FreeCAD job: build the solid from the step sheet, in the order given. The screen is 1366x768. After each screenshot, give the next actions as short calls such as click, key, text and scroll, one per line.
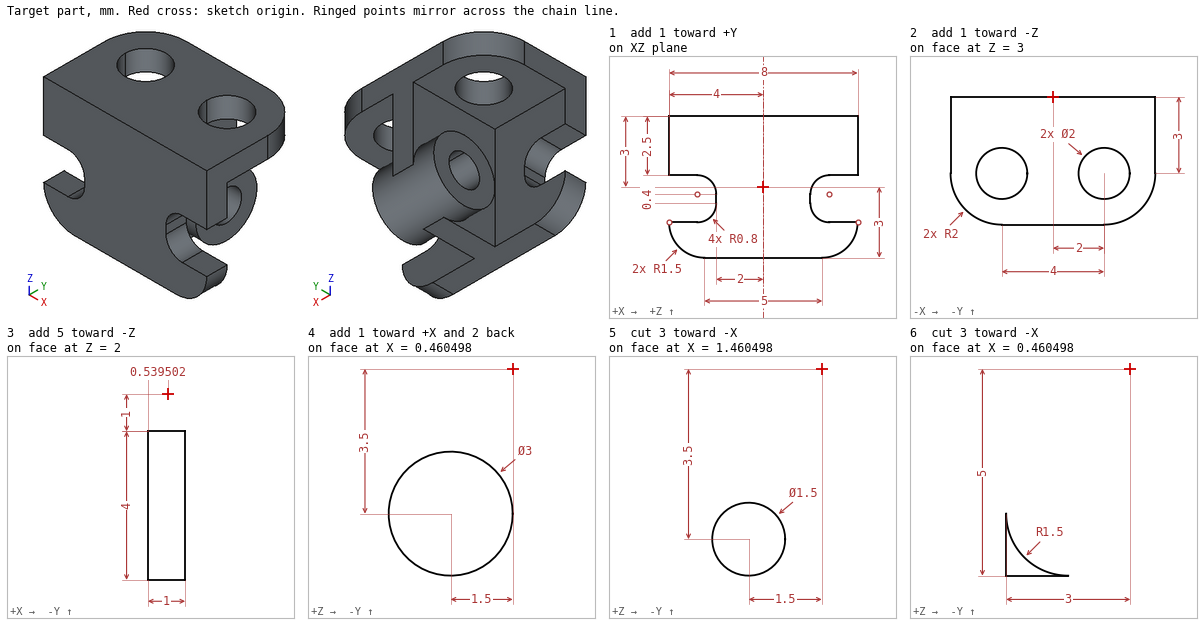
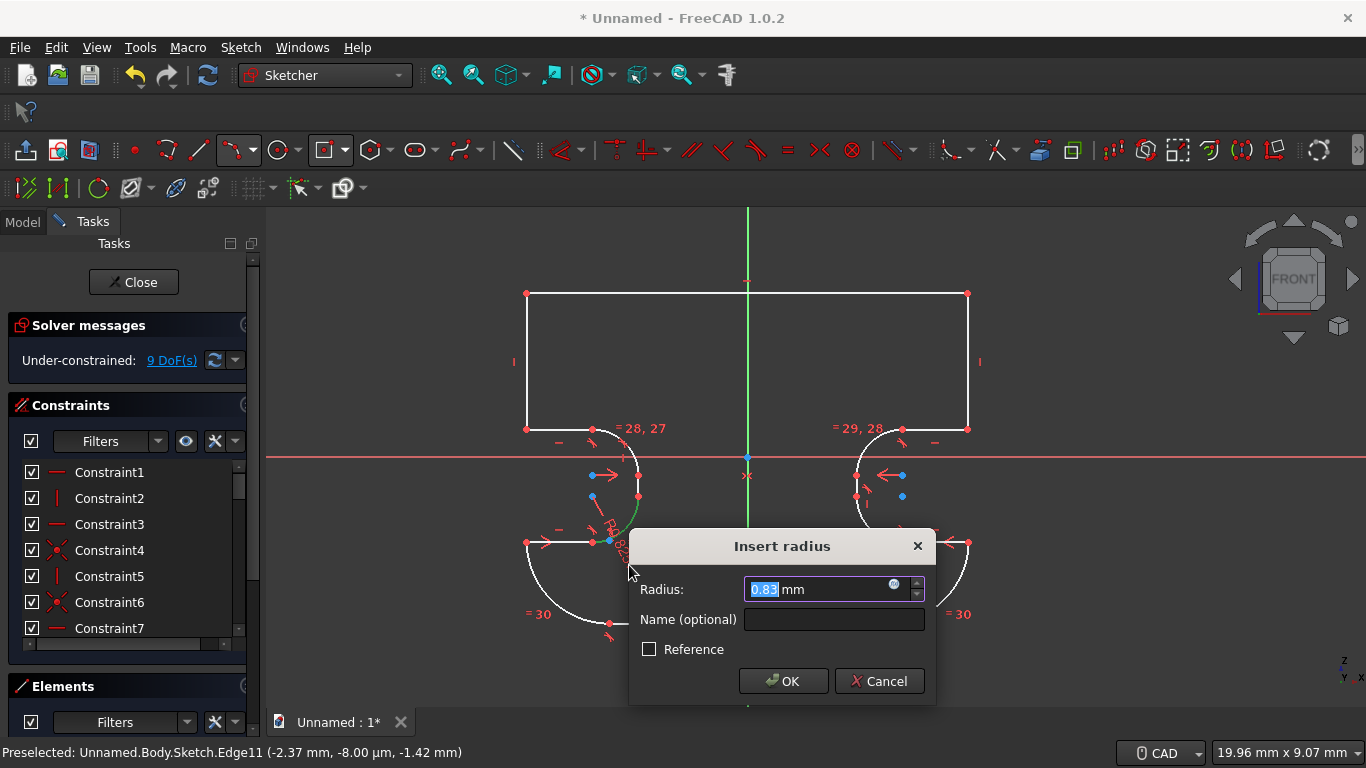
text(0.8)
key(Return)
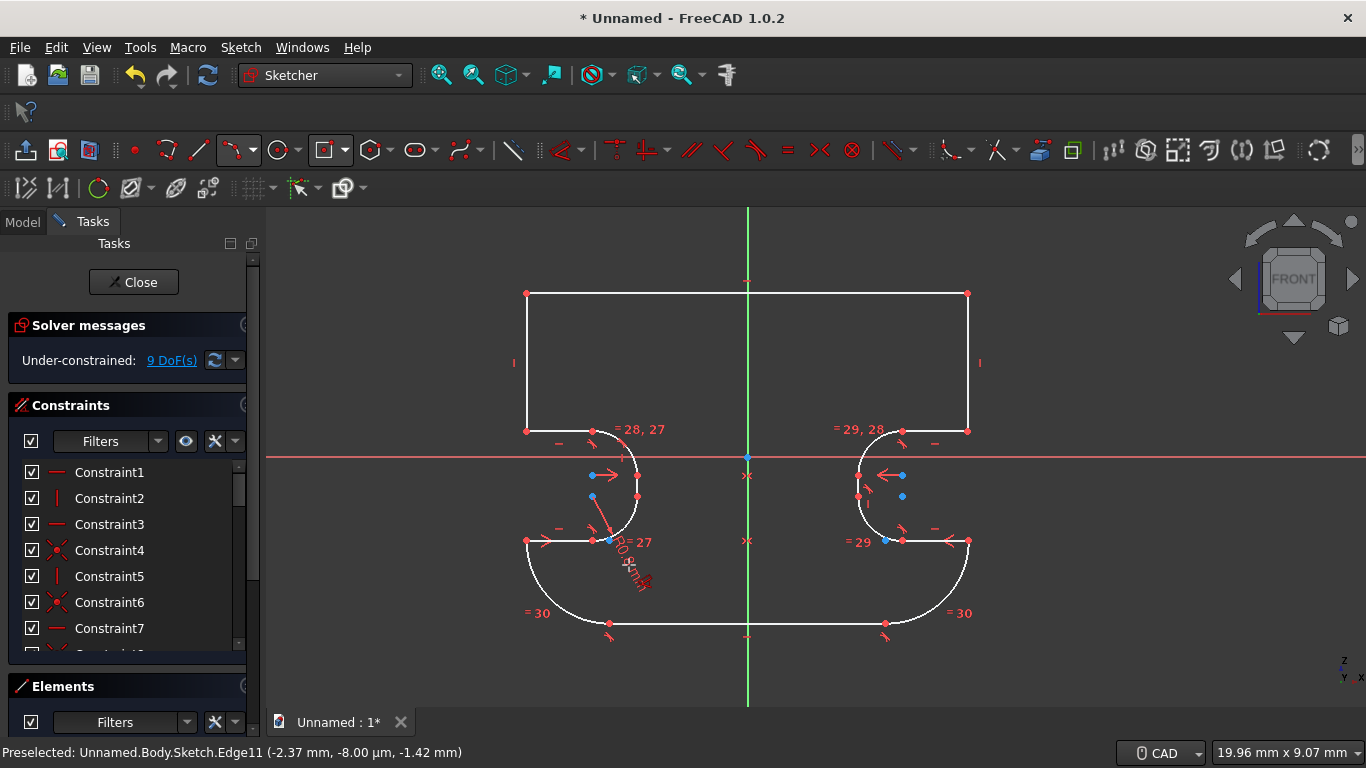
click(923, 615)
click(937, 644)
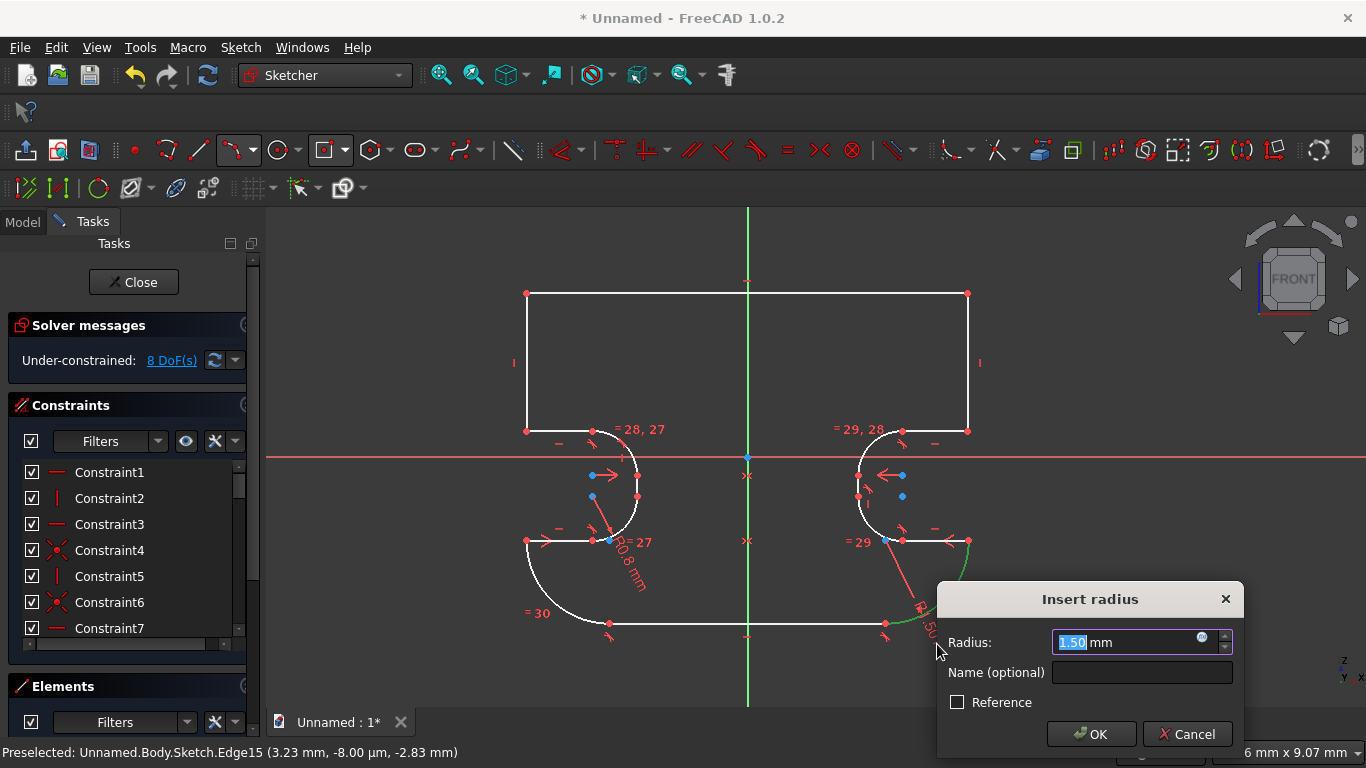
text(1.5)
key(Return)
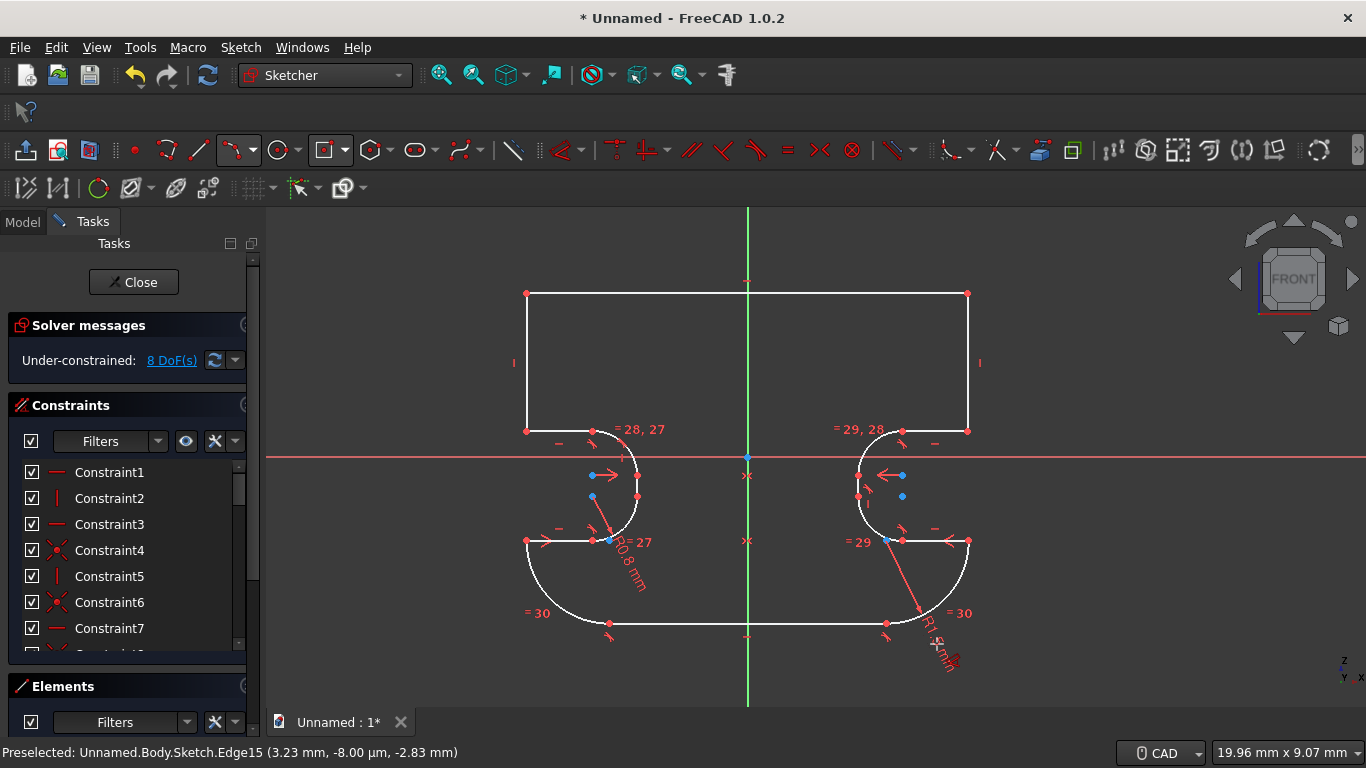
click(659, 293)
click(646, 259)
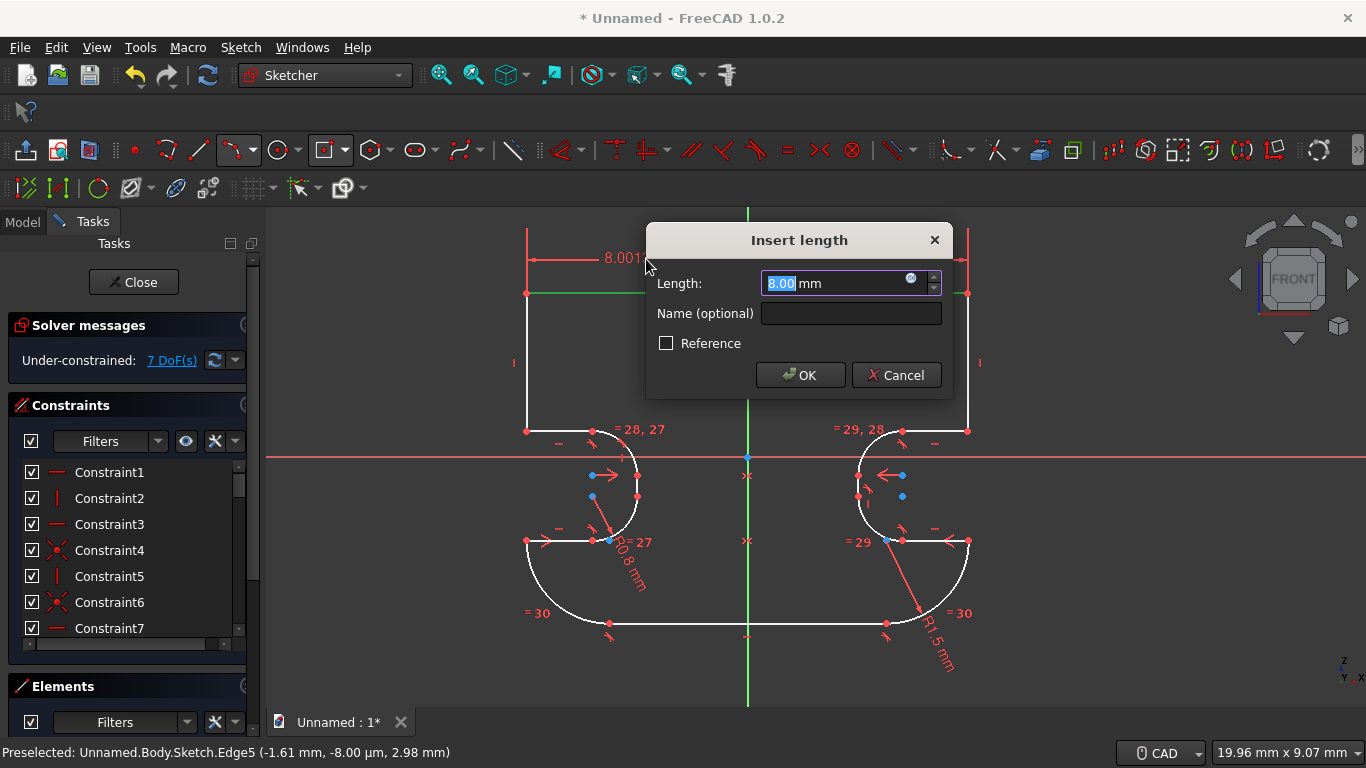
text(8)
key(Return)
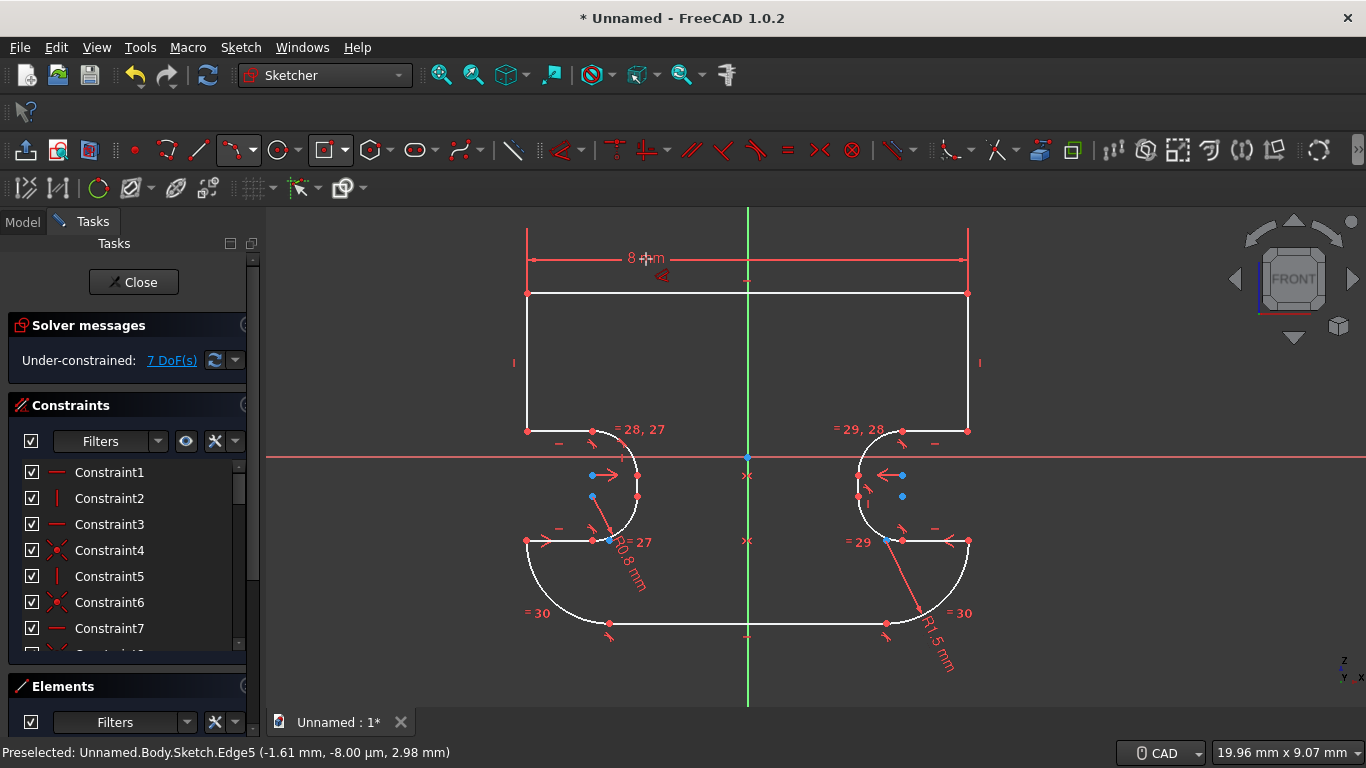
click(803, 624)
click(684, 658)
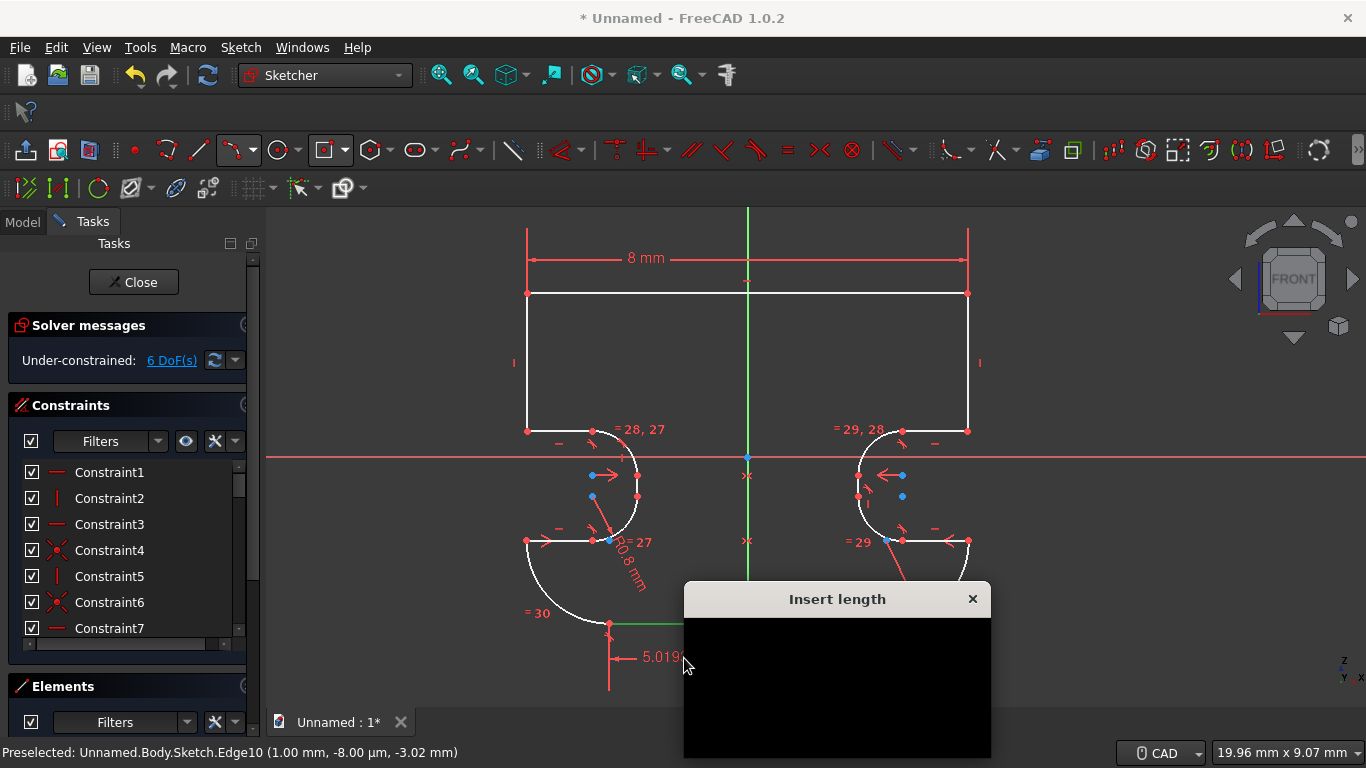
text(5)
key(Return)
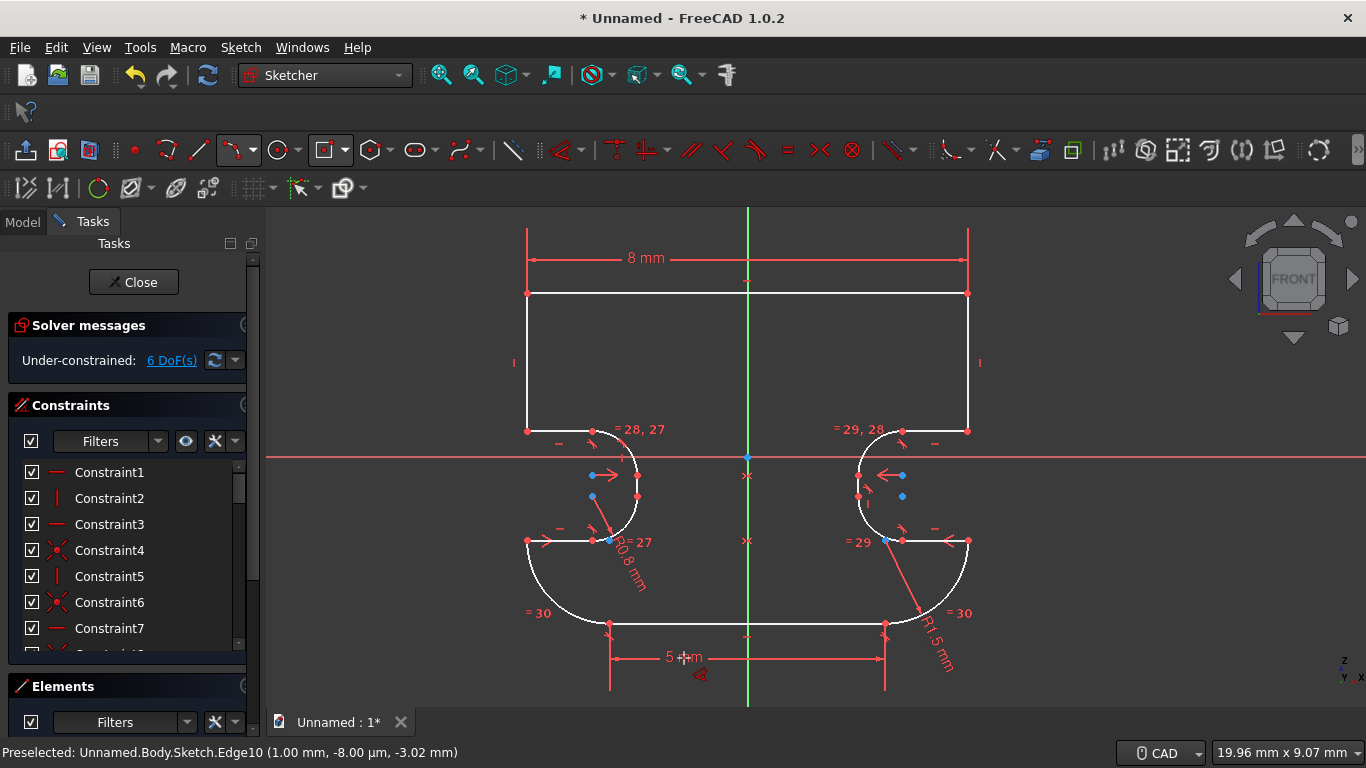
click(637, 497)
click(692, 531)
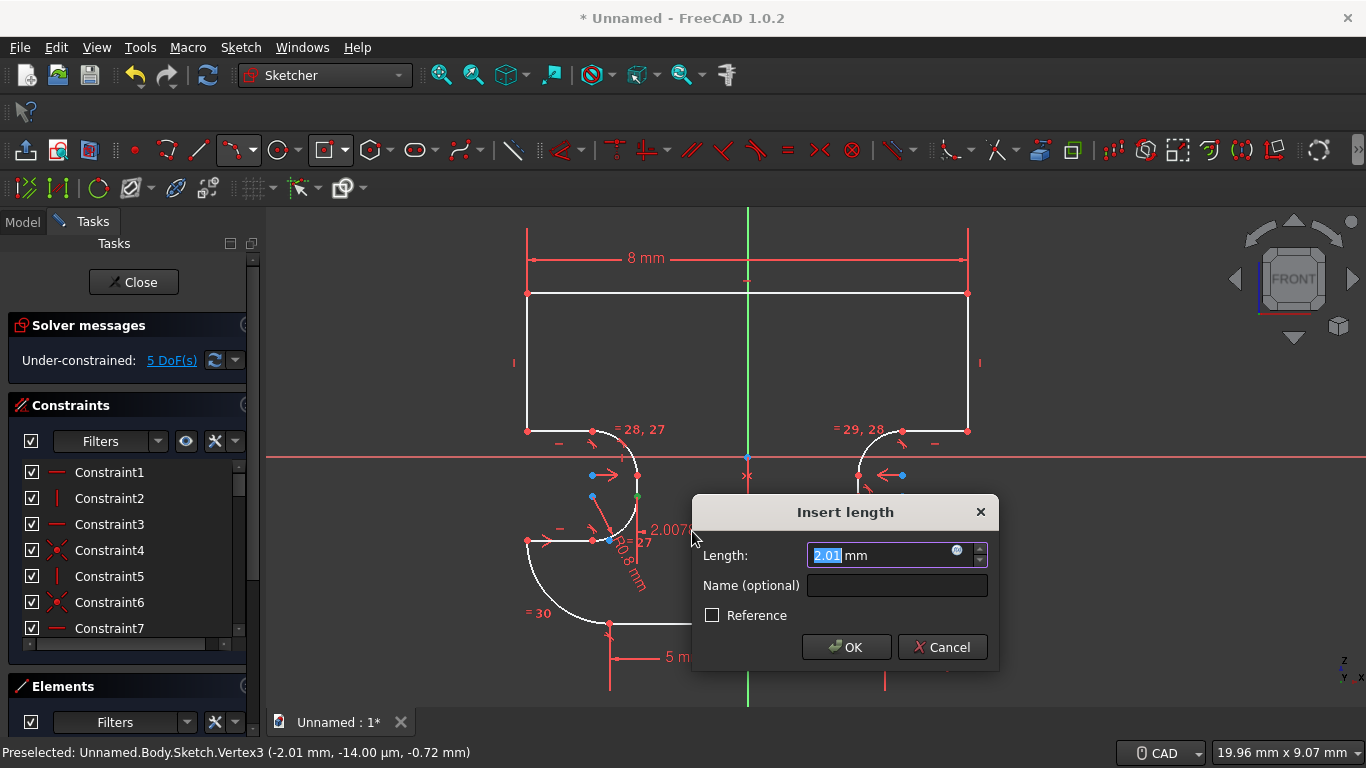
text(2)
key(Return)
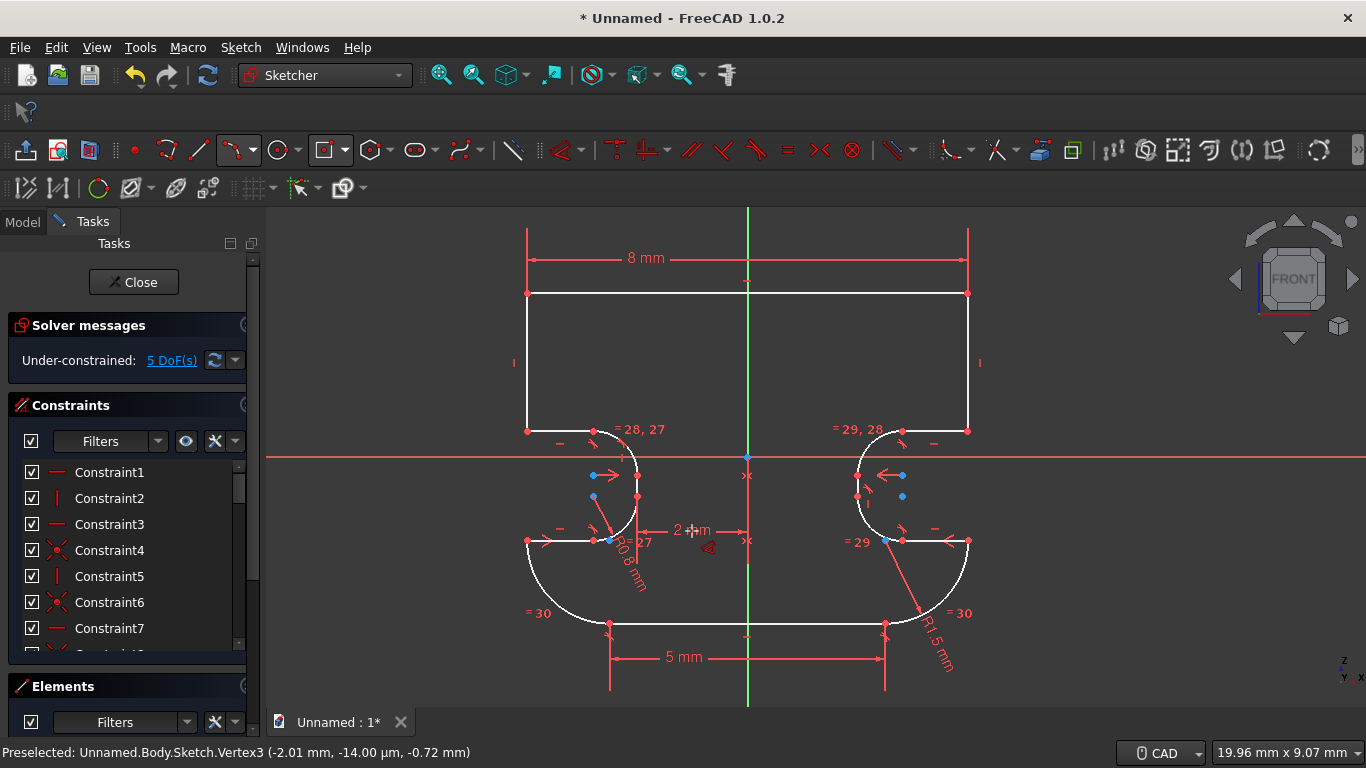
click(527, 431)
click(637, 397)